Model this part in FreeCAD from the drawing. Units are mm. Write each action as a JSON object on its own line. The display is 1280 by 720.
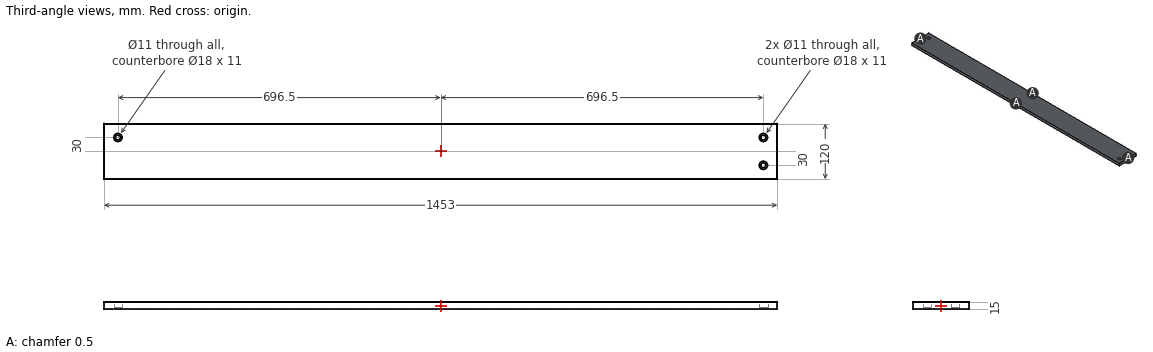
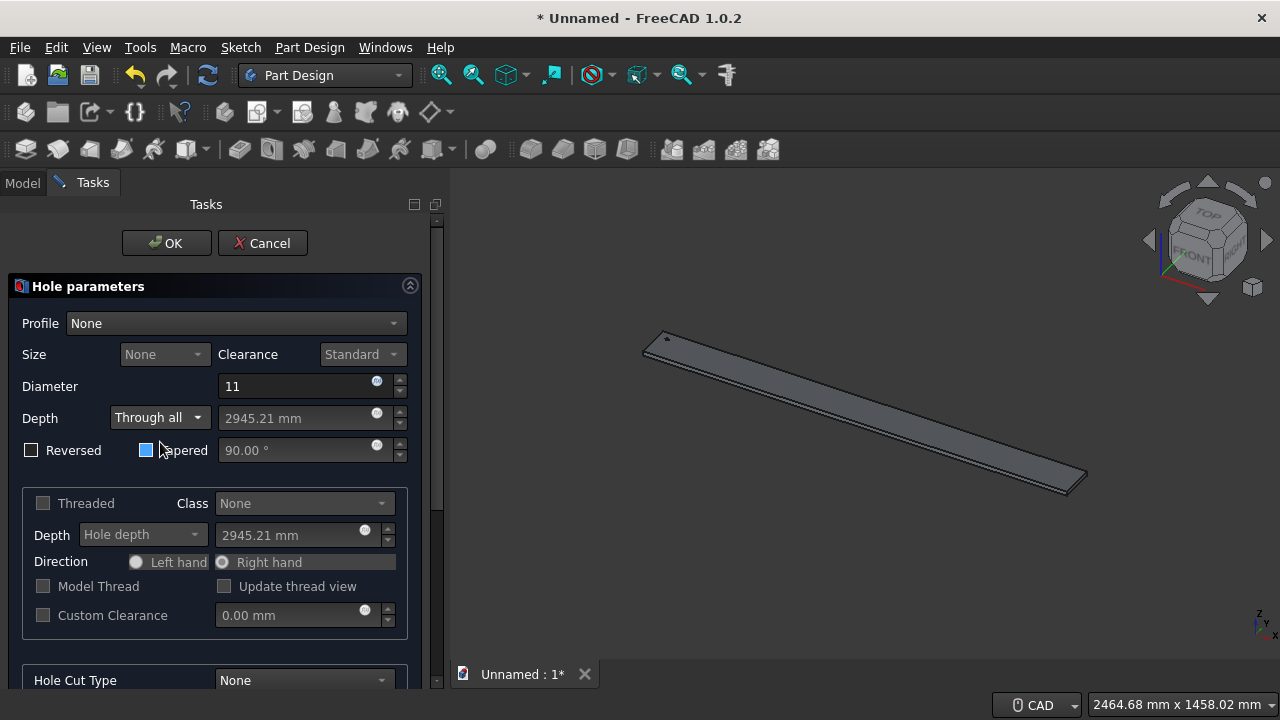
{"action": "scroll", "coordinate": [437, 451], "scroll_direction": "down", "scroll_amount": 2}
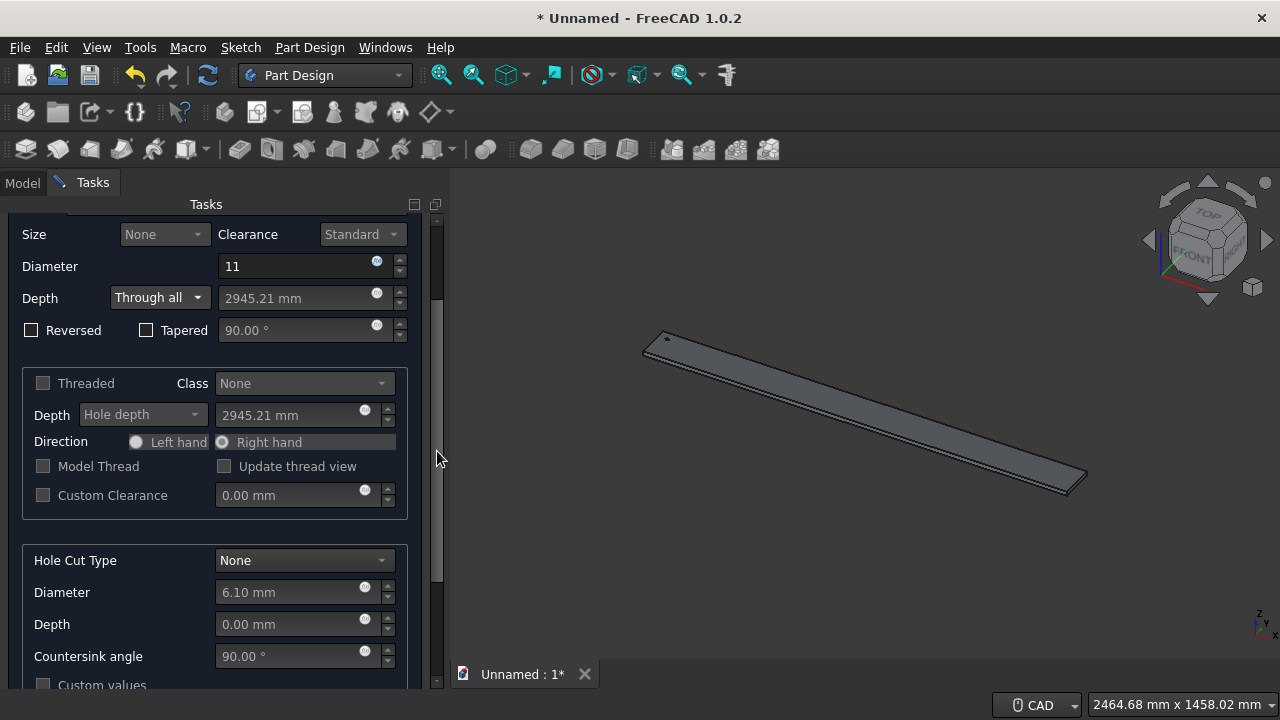
{"action": "left_click", "coordinate": [306, 560]}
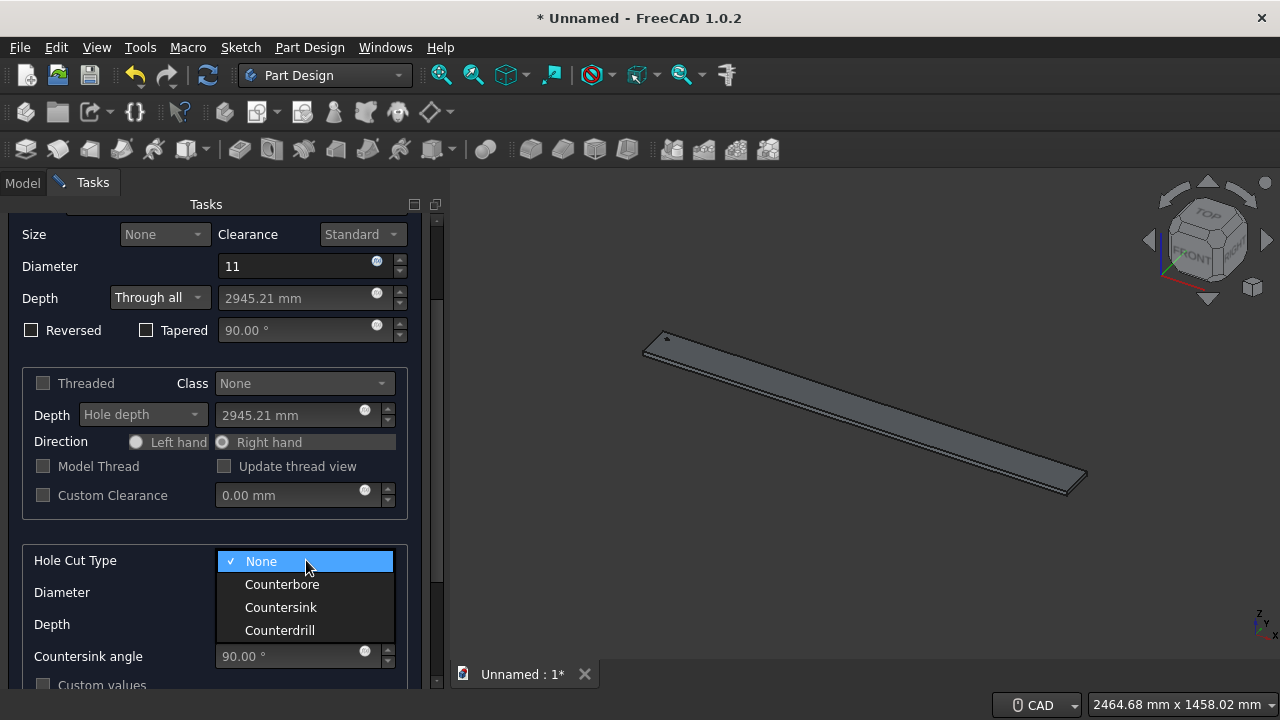
{"action": "left_click", "coordinate": [304, 584]}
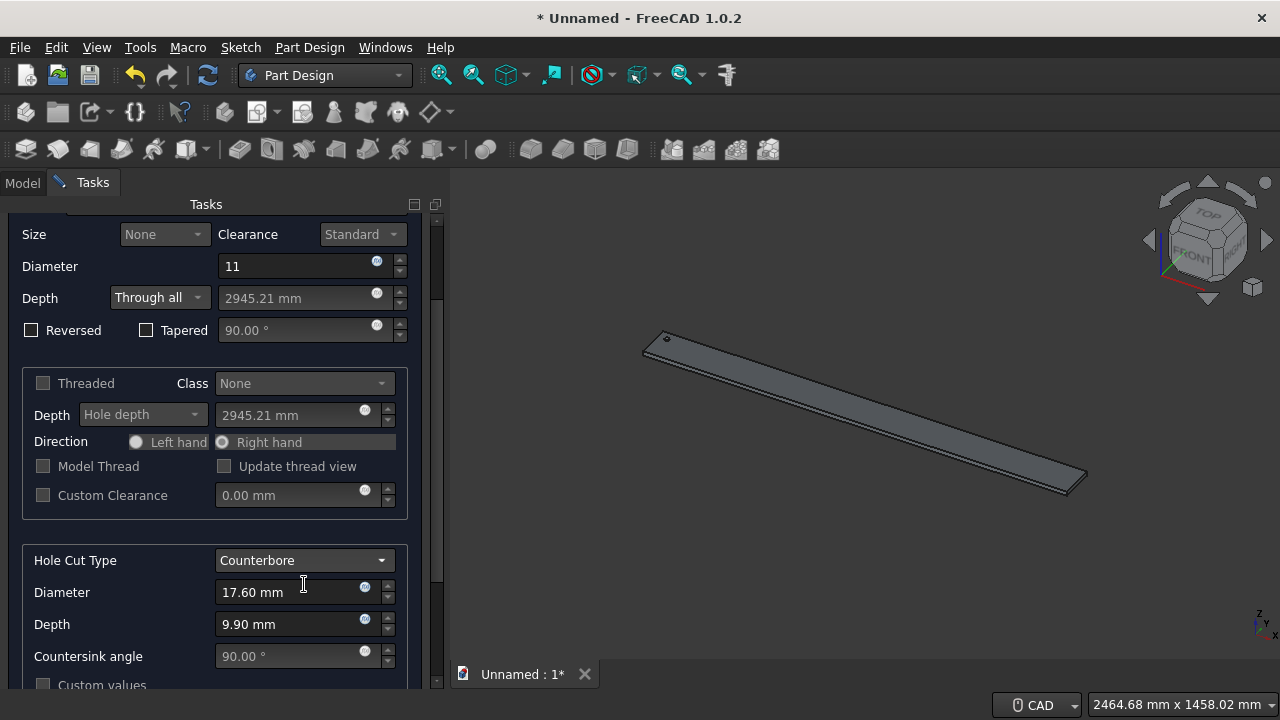
{"action": "triple_click", "coordinate": [298, 592]}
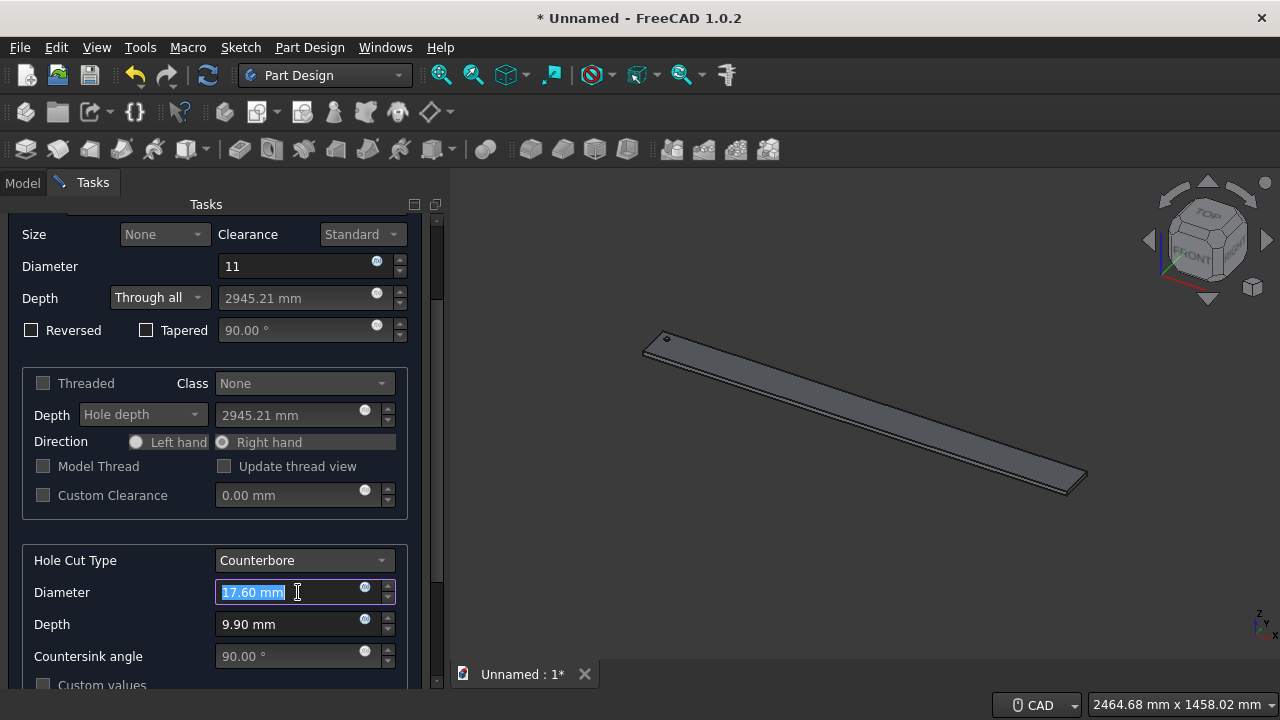
{"action": "type", "text": "18"}
{"action": "key", "text": "Tab"}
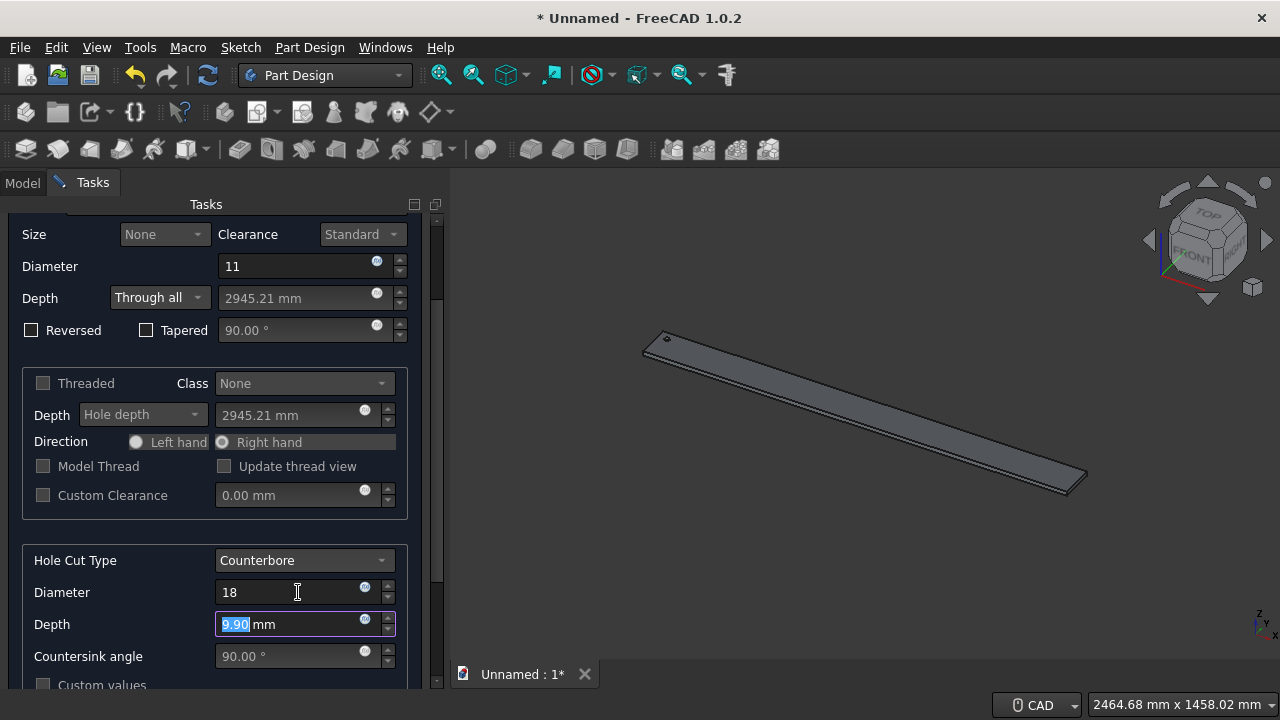
{"action": "type", "text": "11"}
{"action": "key", "text": "Tab"}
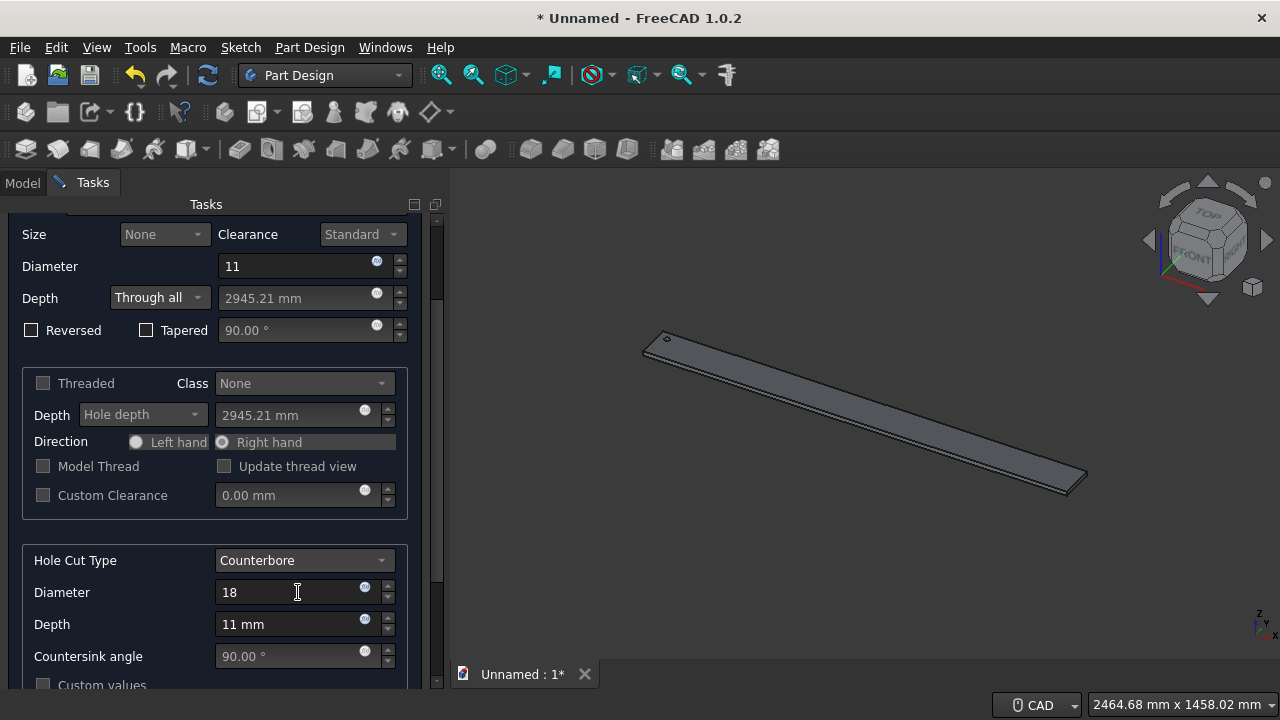
{"action": "scroll", "coordinate": [437, 451], "scroll_direction": "up", "scroll_amount": 3}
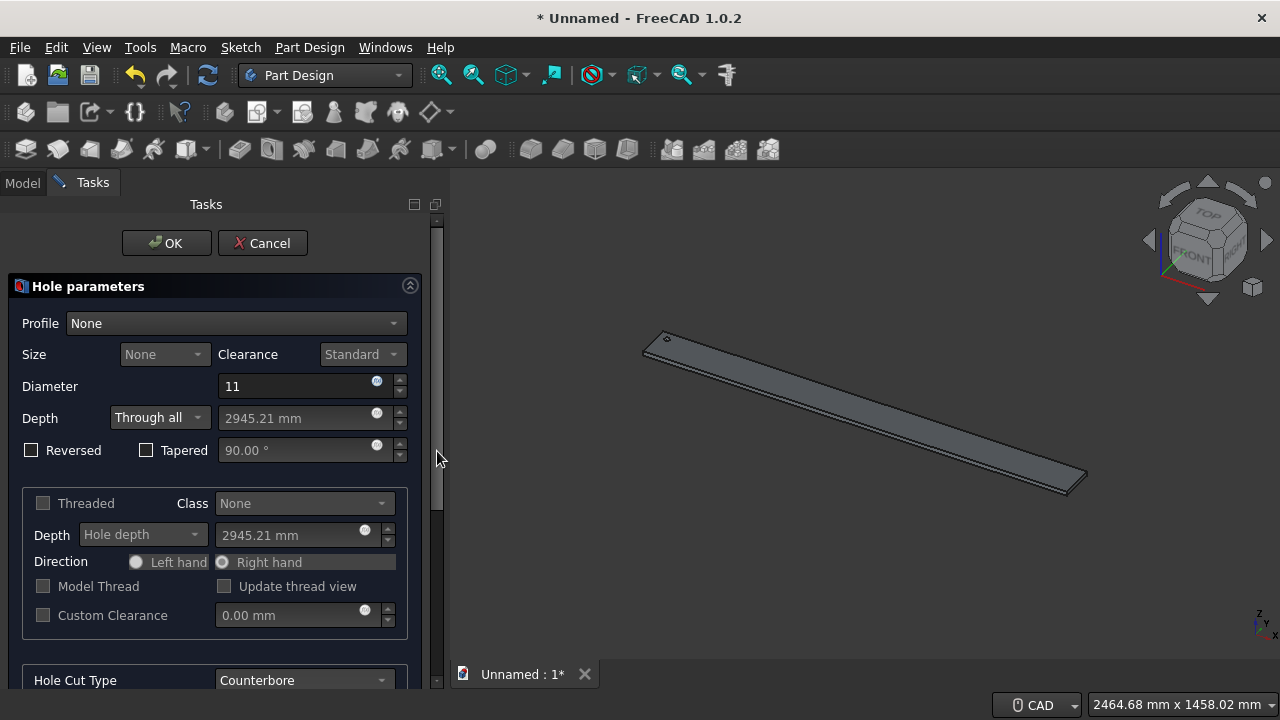
{"action": "left_click", "coordinate": [167, 243]}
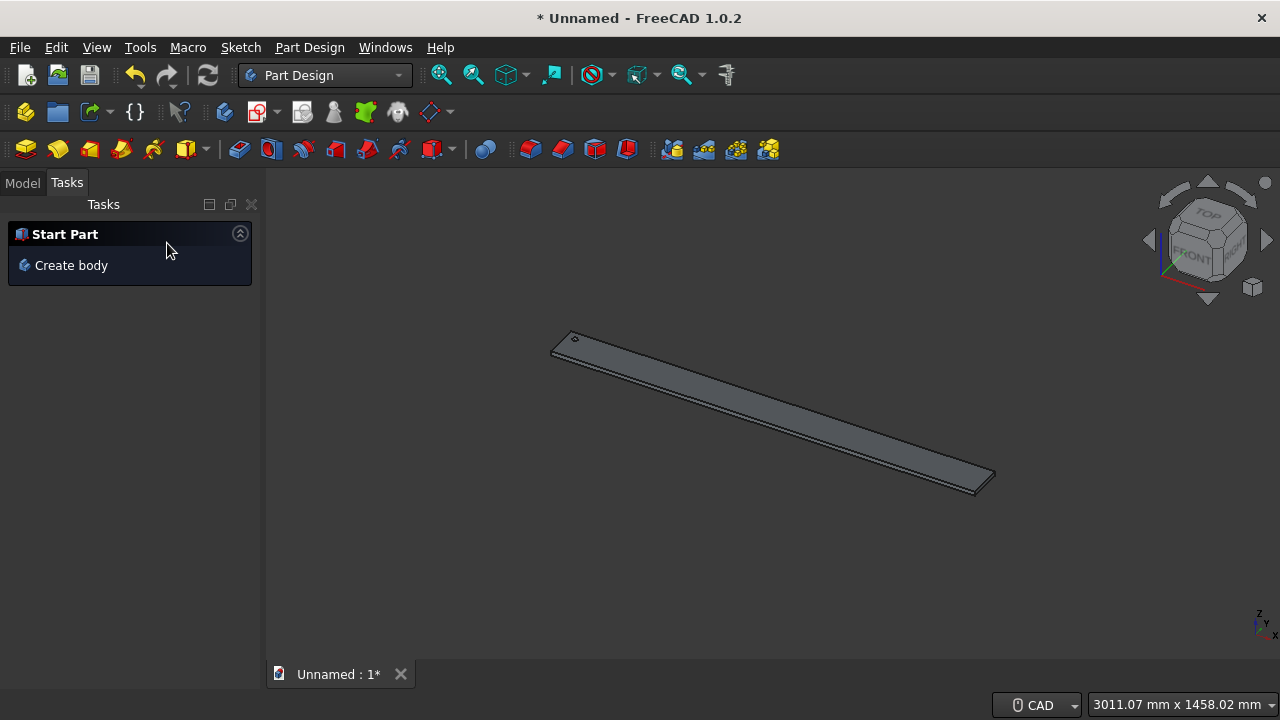
{"action": "left_click", "coordinate": [442, 76]}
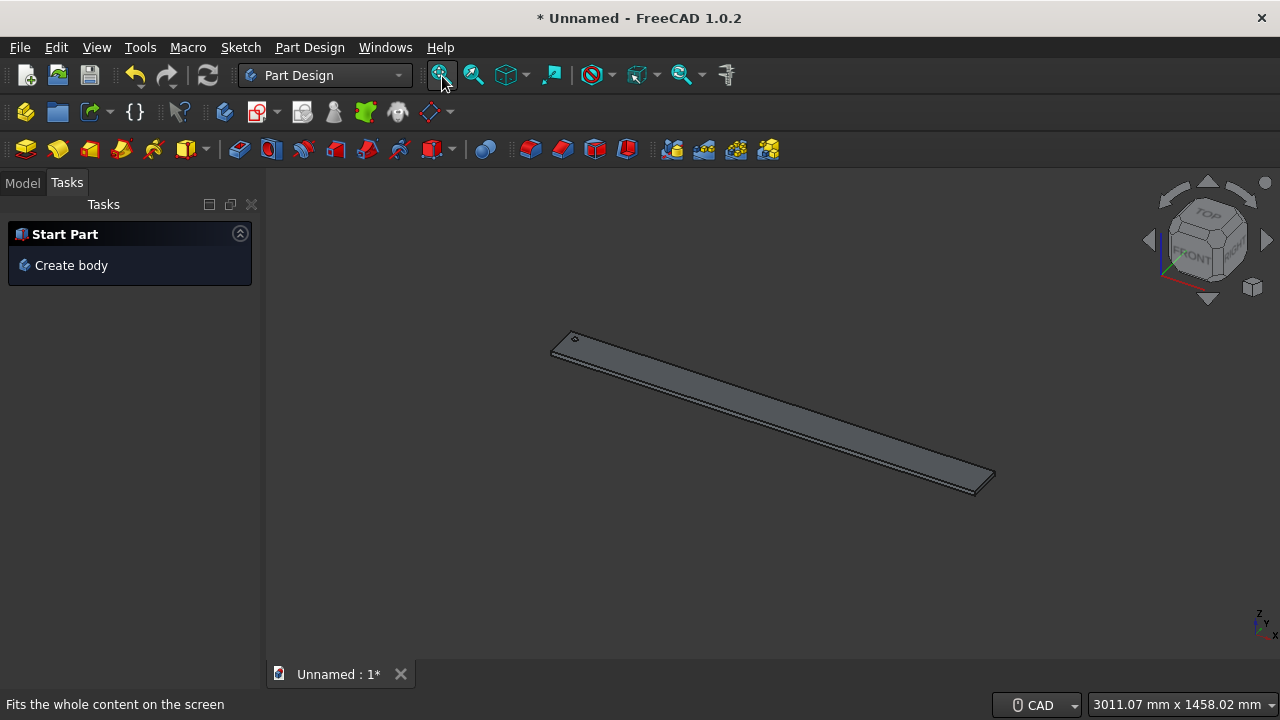
{"action": "left_click", "coordinate": [955, 471]}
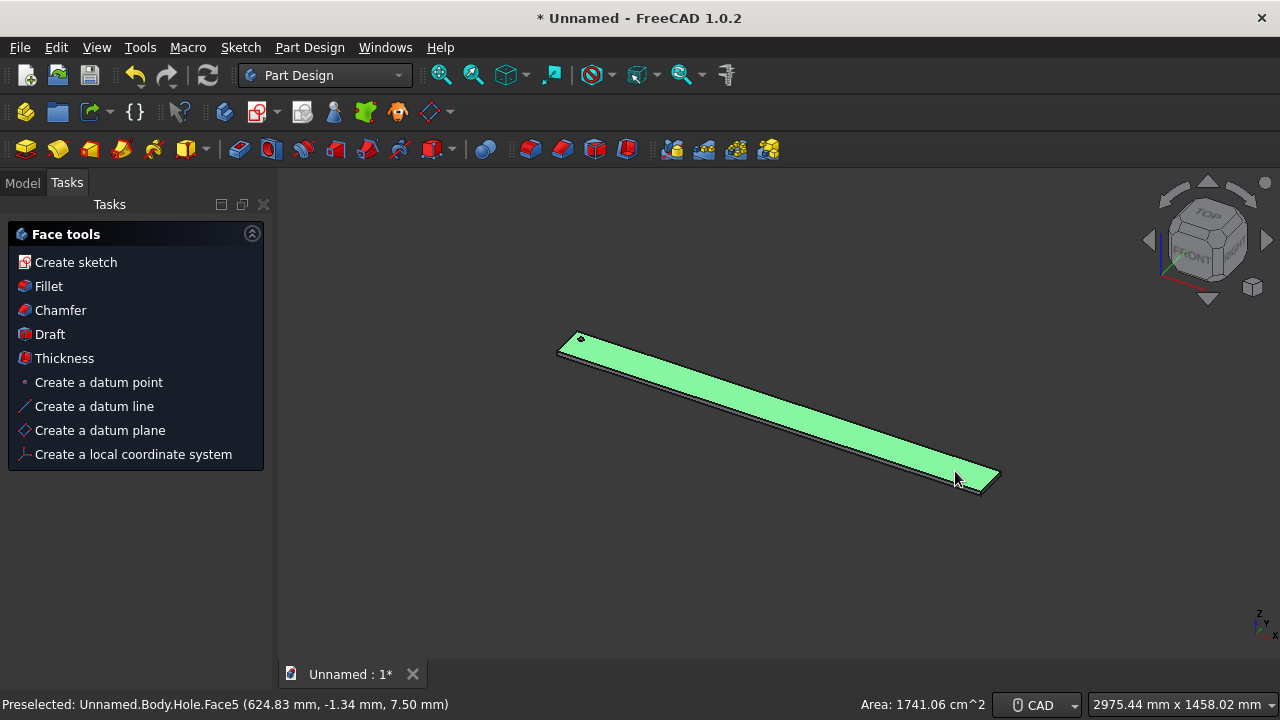
{"action": "left_click", "coordinate": [258, 112]}